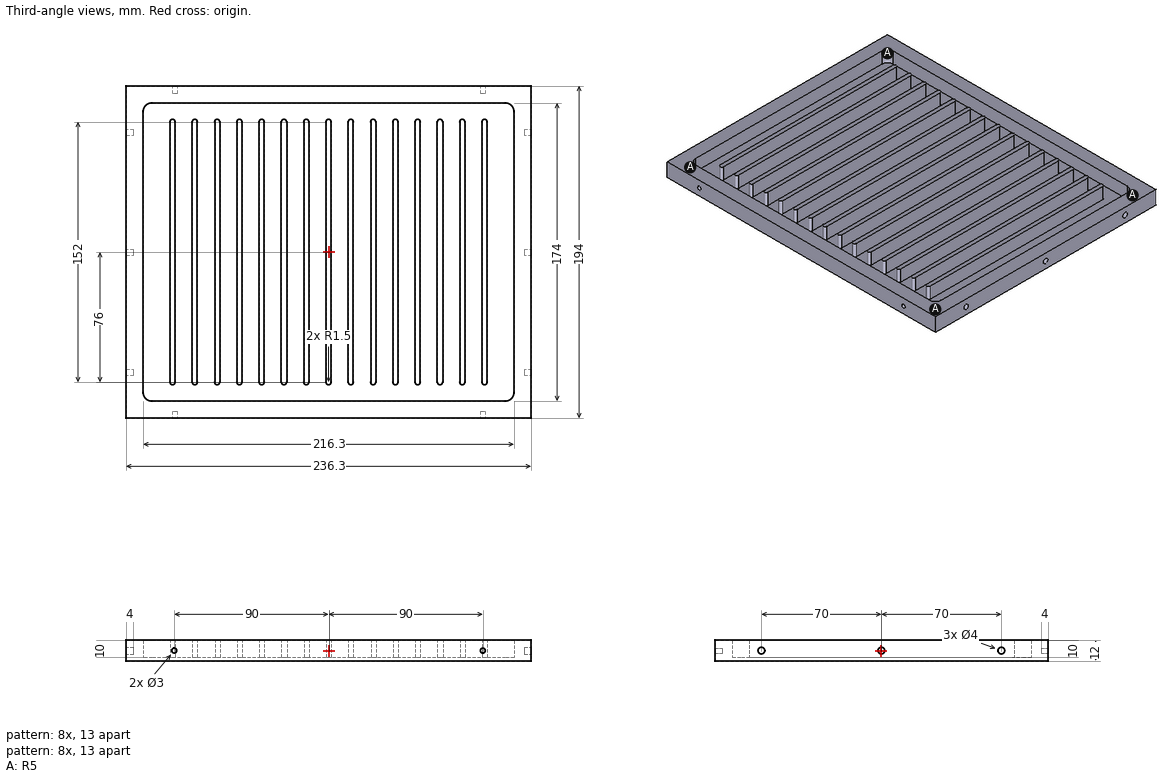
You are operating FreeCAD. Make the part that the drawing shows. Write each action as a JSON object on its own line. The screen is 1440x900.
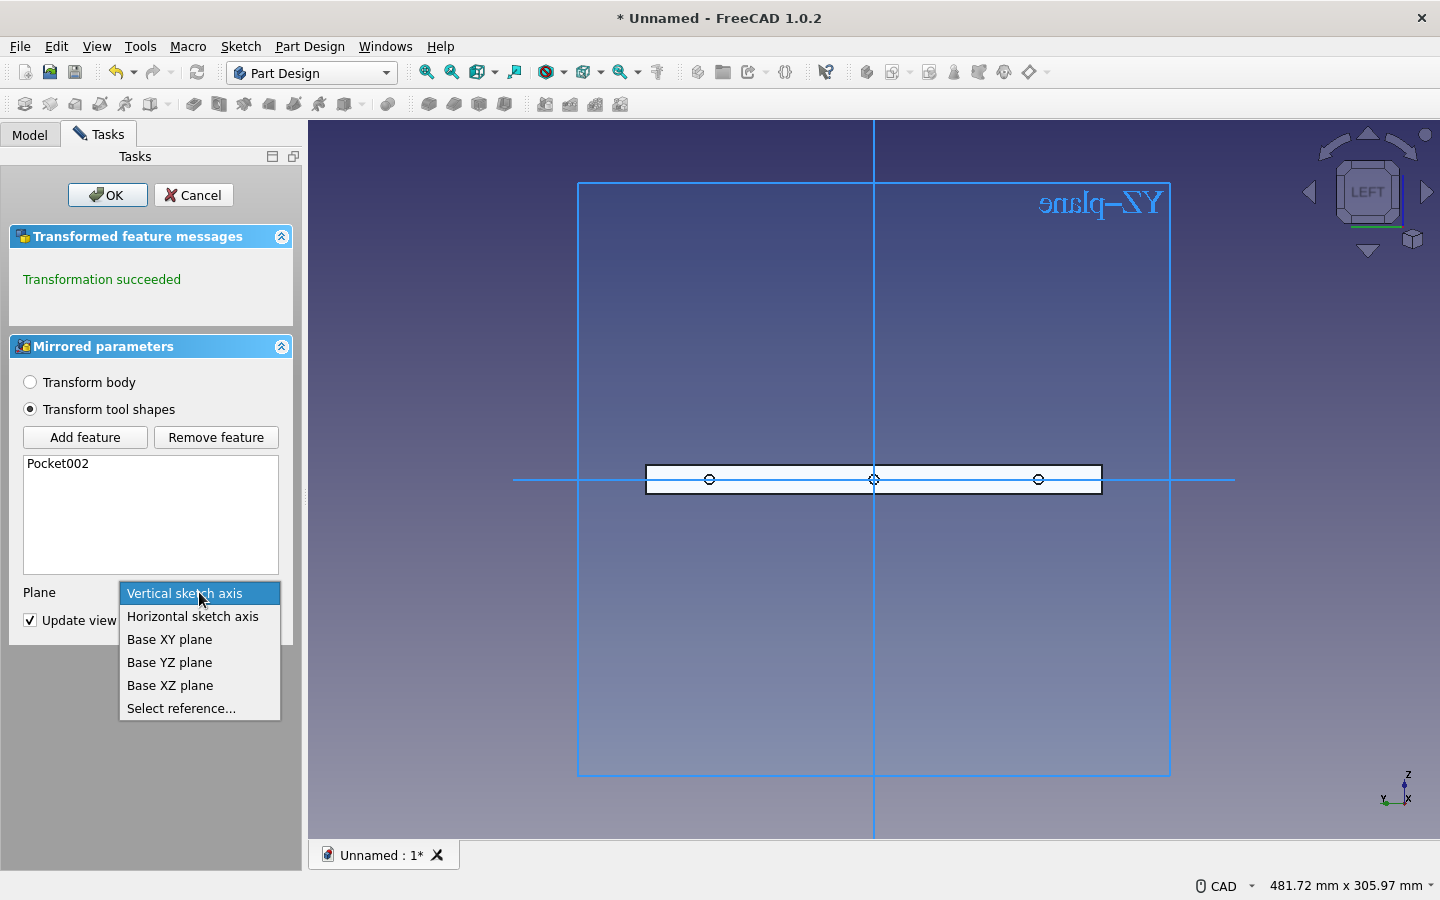
{"action": "left_click", "coordinate": [198, 662]}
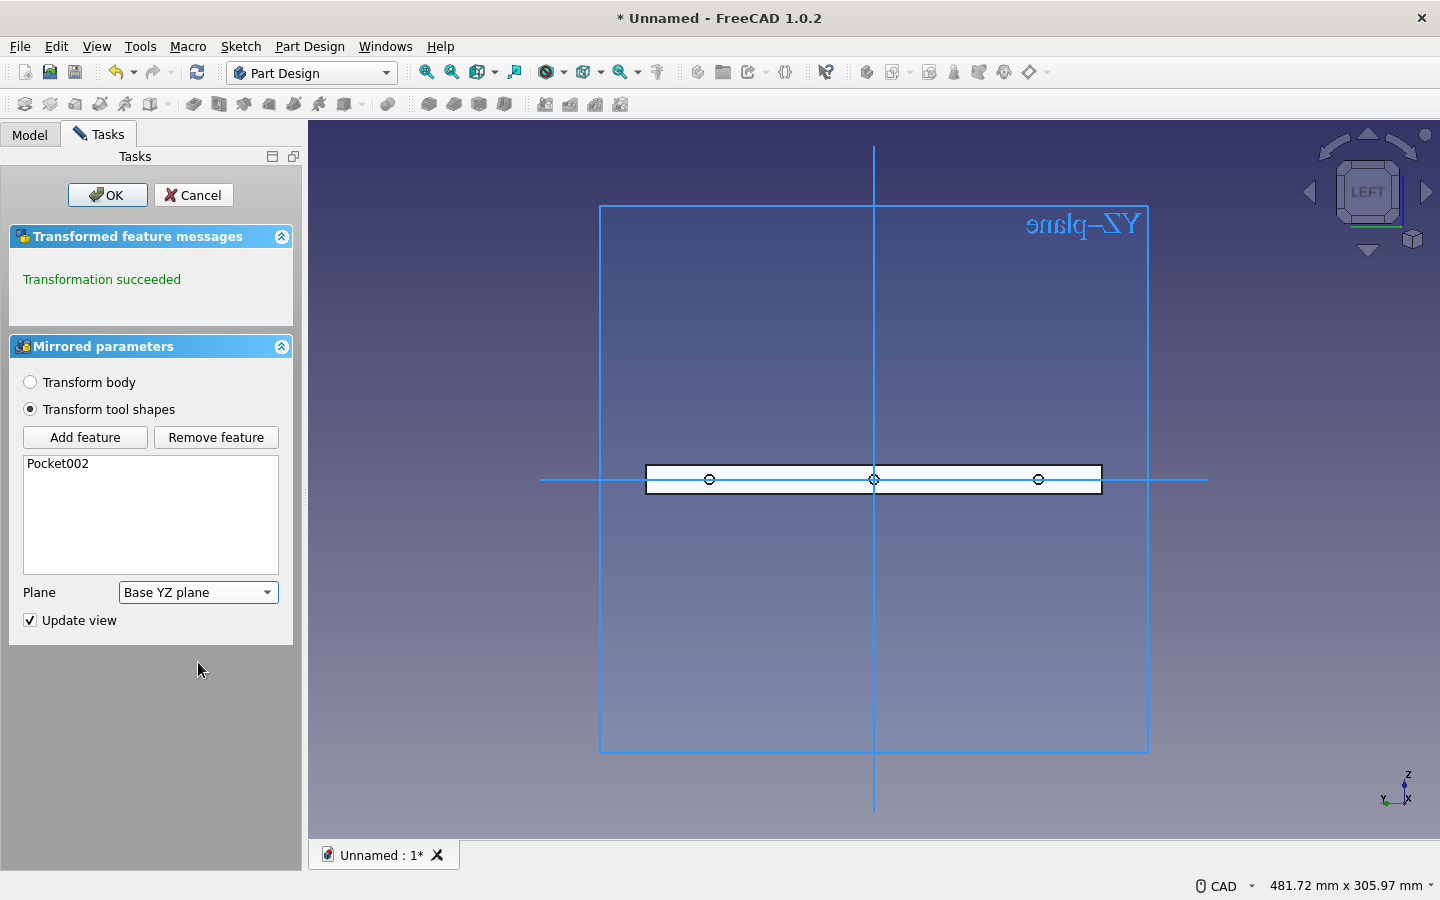
{"action": "left_click", "coordinate": [108, 195]}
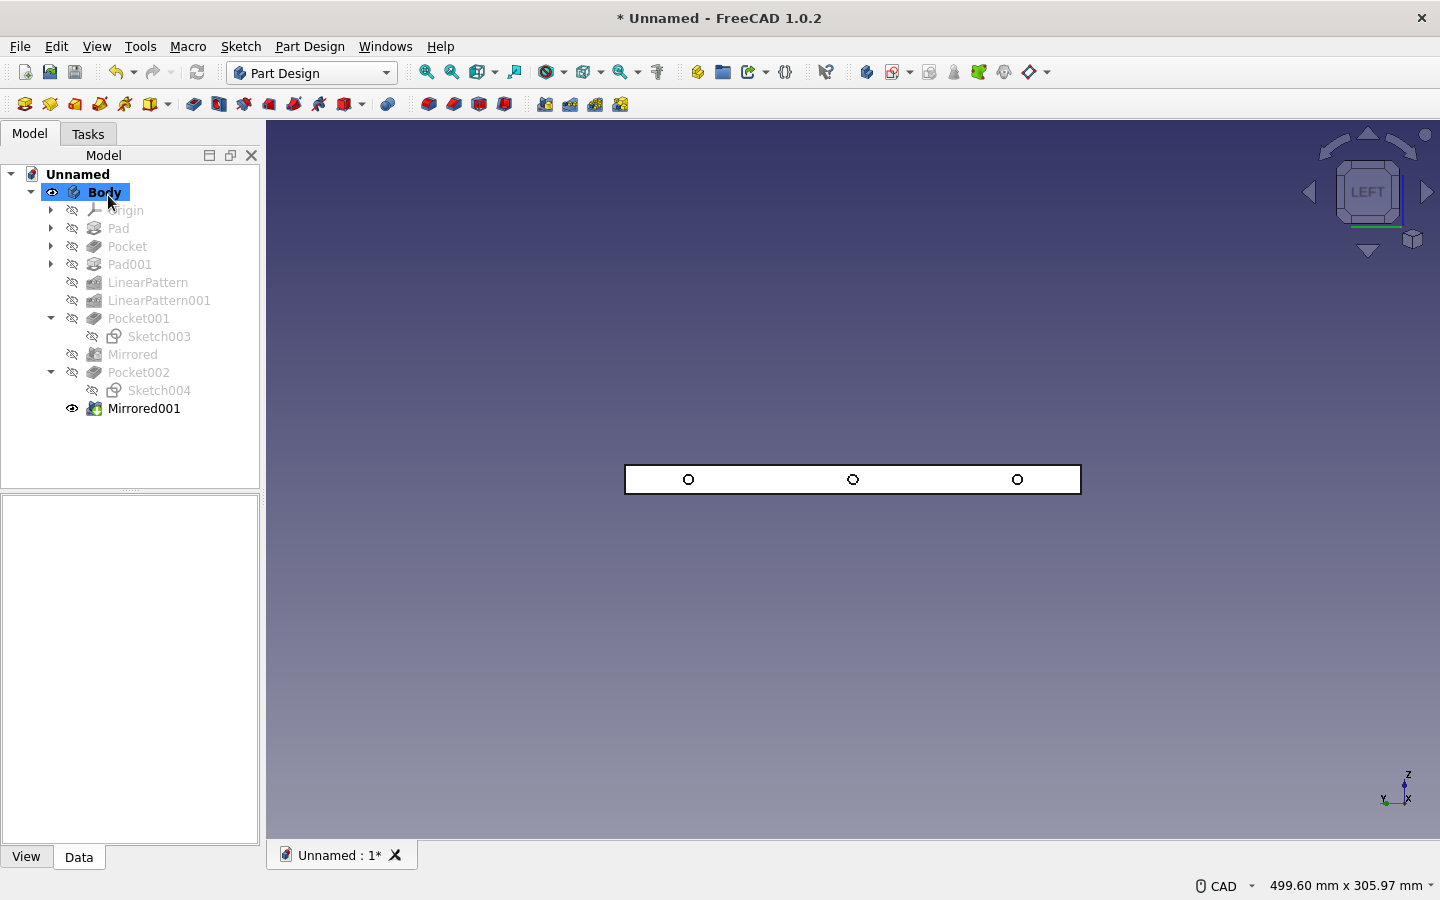
{"action": "left_click", "coordinate": [427, 72]}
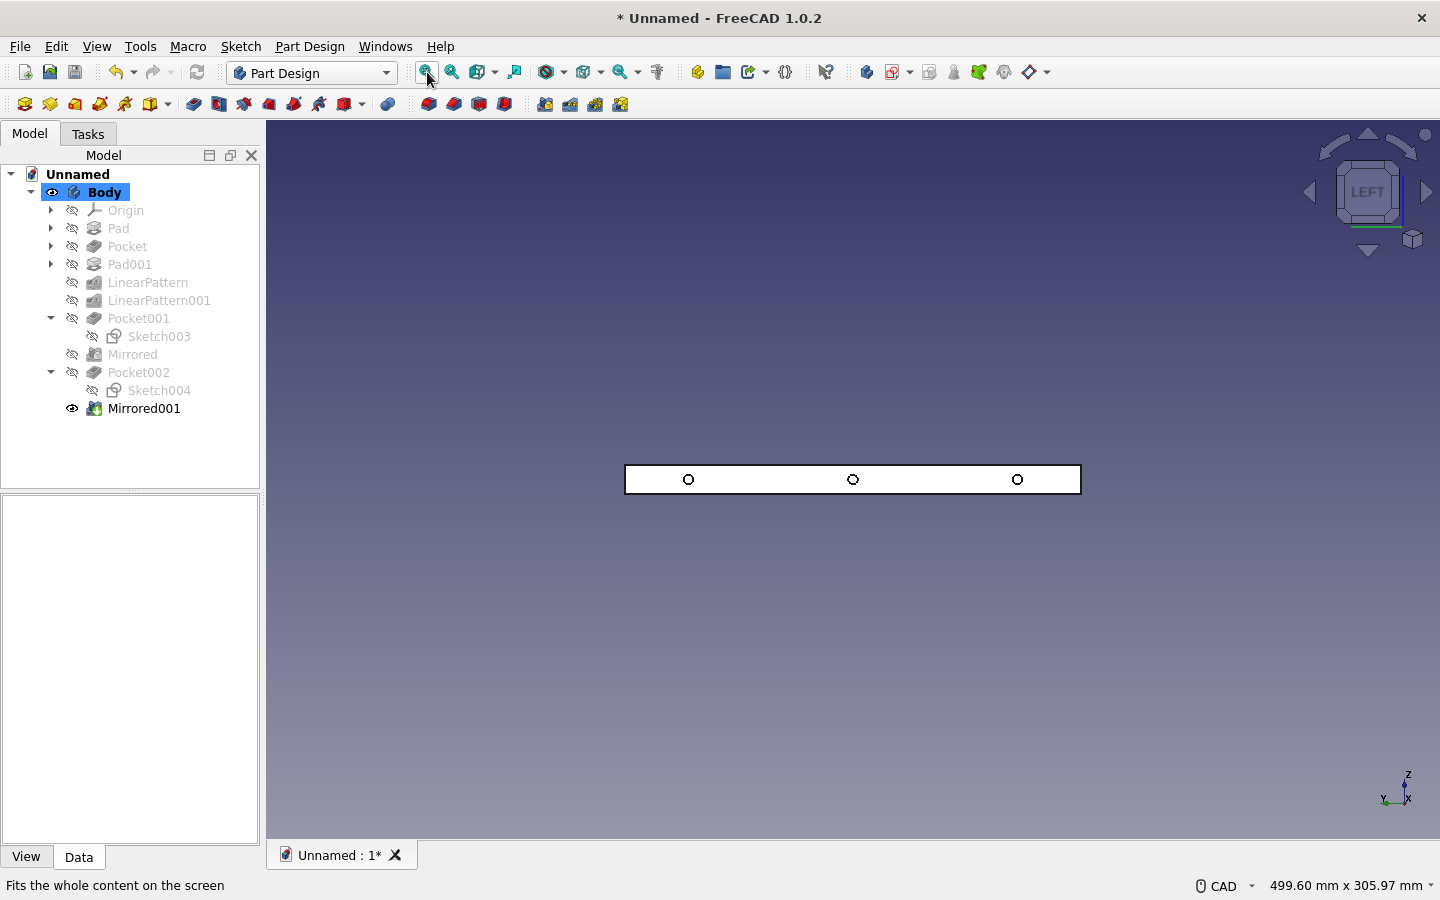
{"action": "key", "text": "0"}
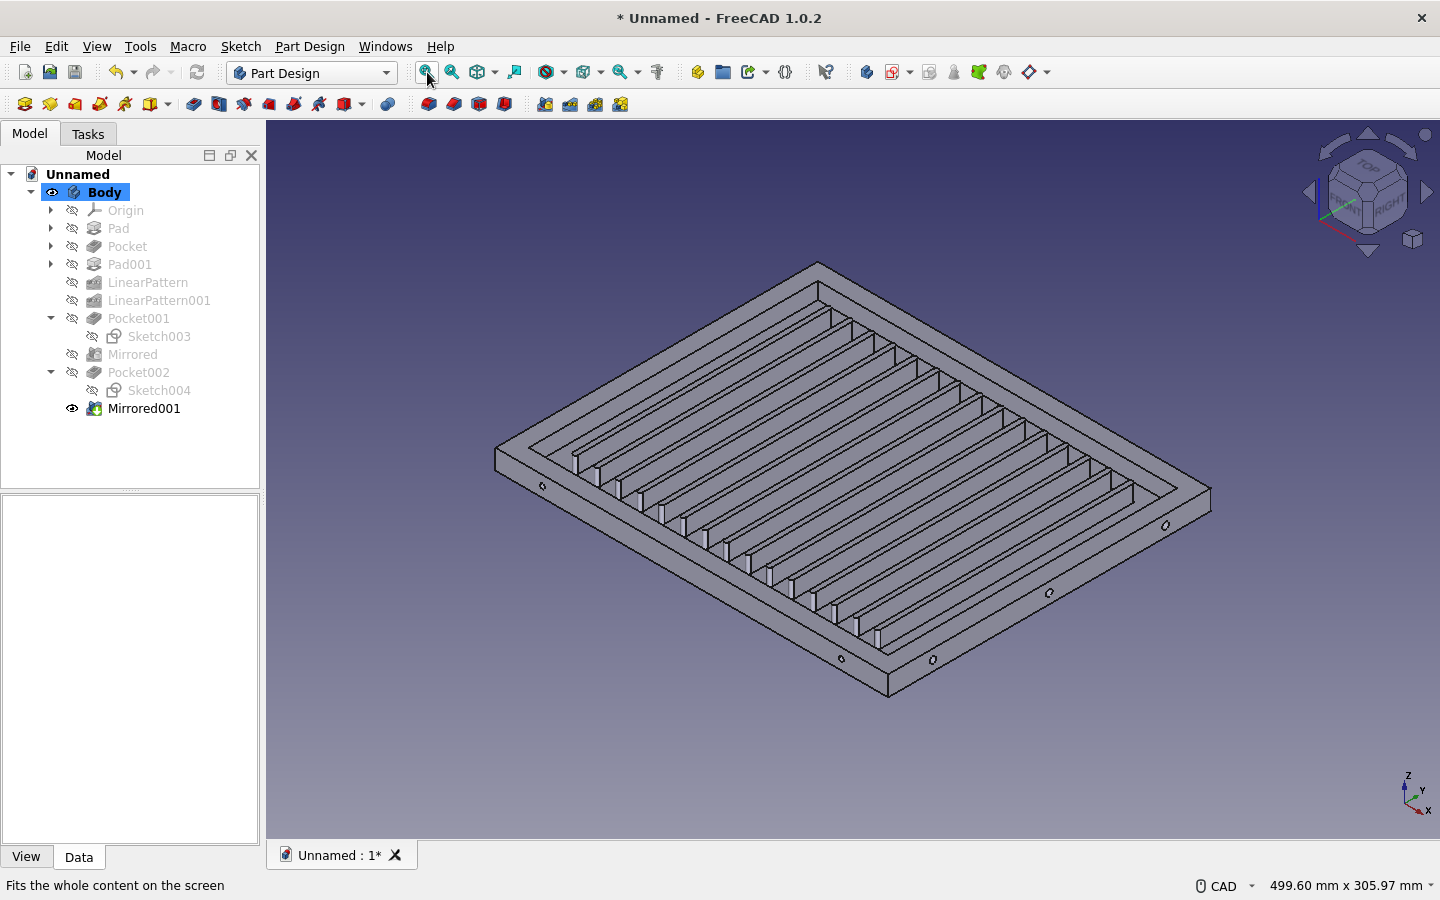
{"action": "key", "text": "2"}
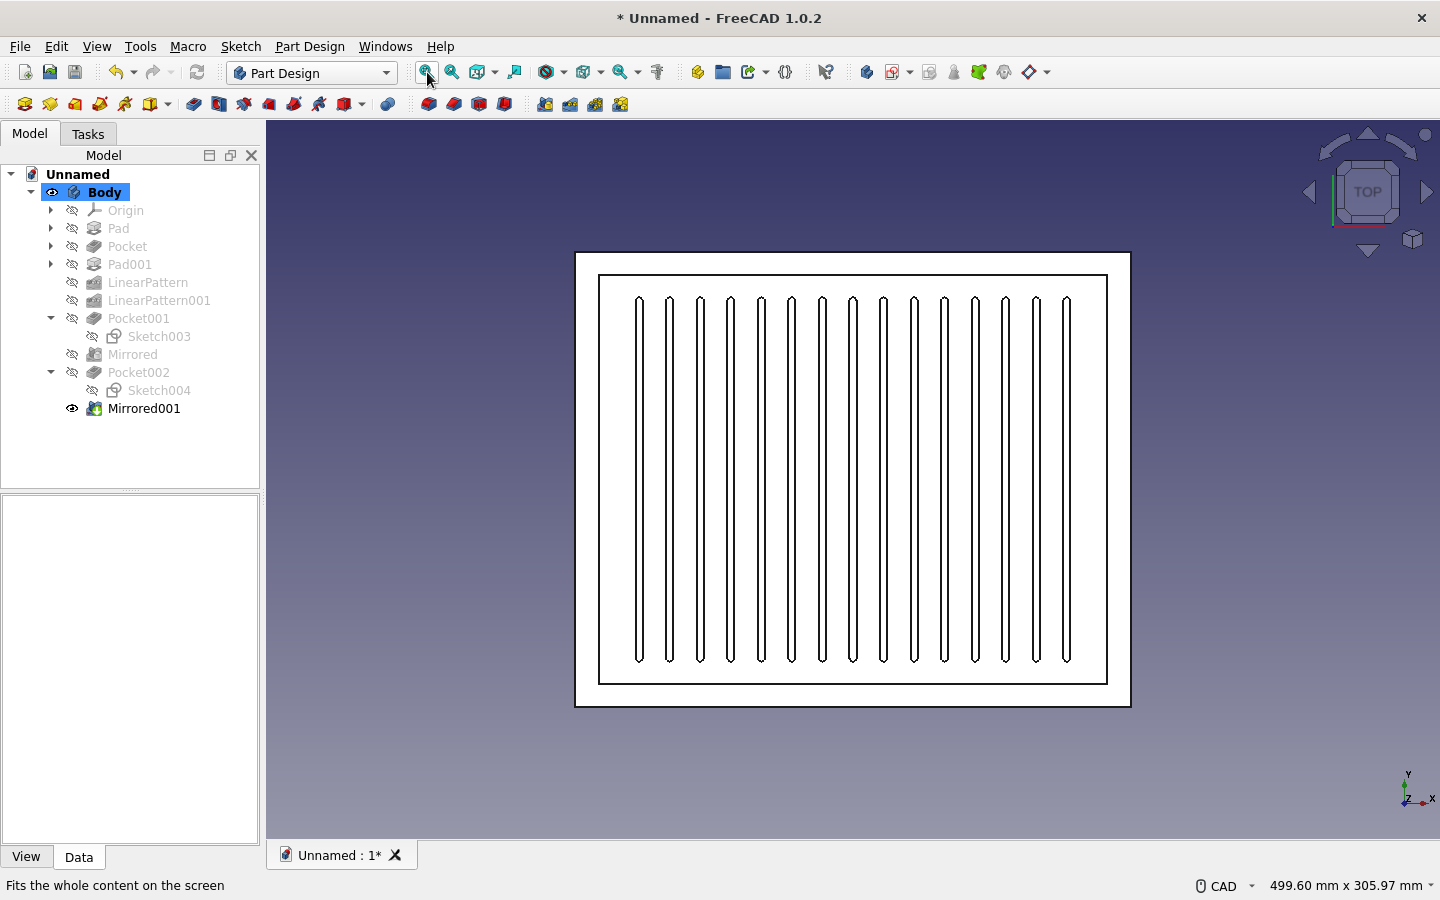
{"action": "key", "text": "1"}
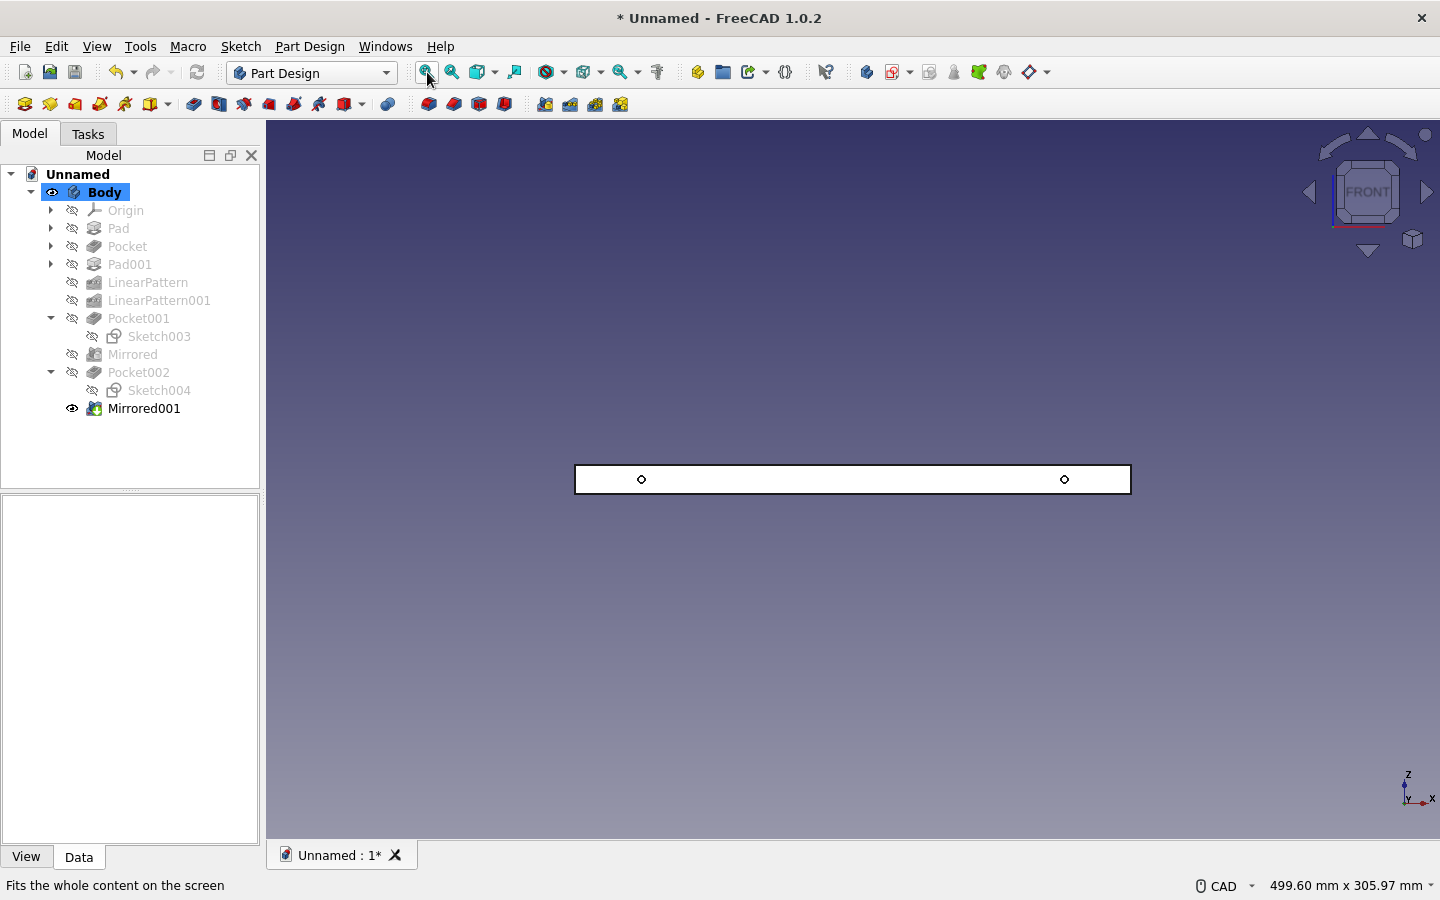
{"action": "key", "text": "3"}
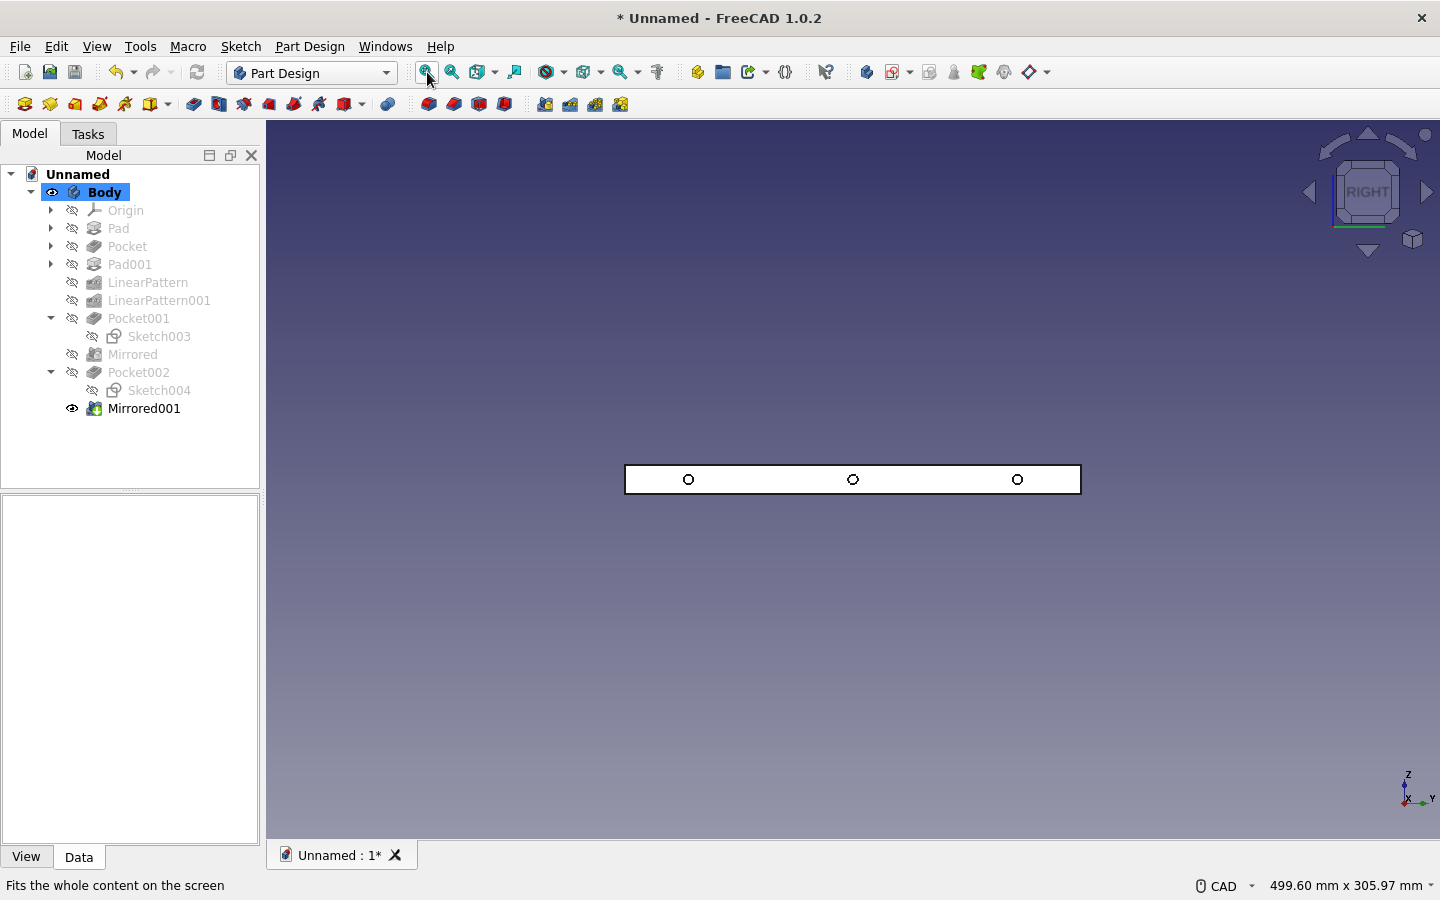
{"action": "left_click", "coordinate": [427, 72]}